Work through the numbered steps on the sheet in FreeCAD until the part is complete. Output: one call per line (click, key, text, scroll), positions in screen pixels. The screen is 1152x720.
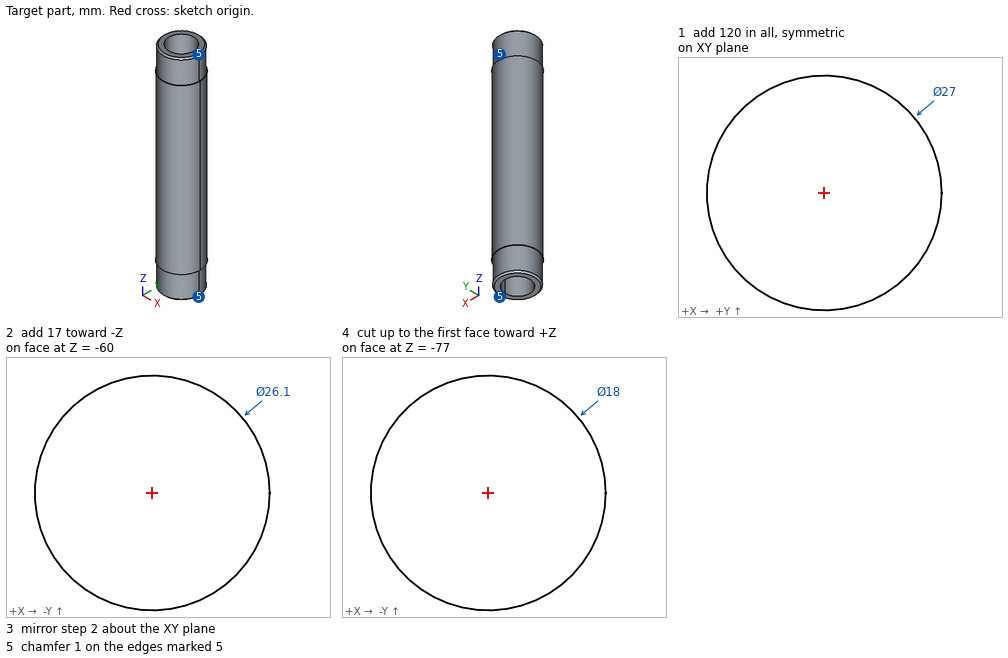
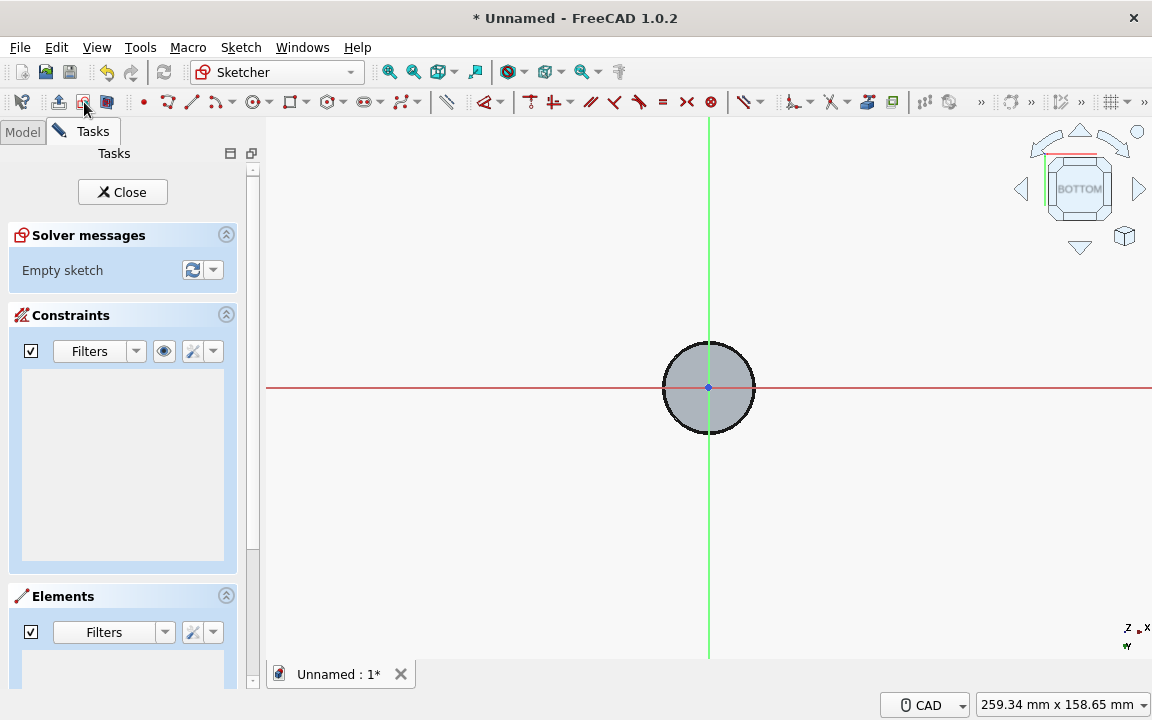
scroll(722, 388, up, 9)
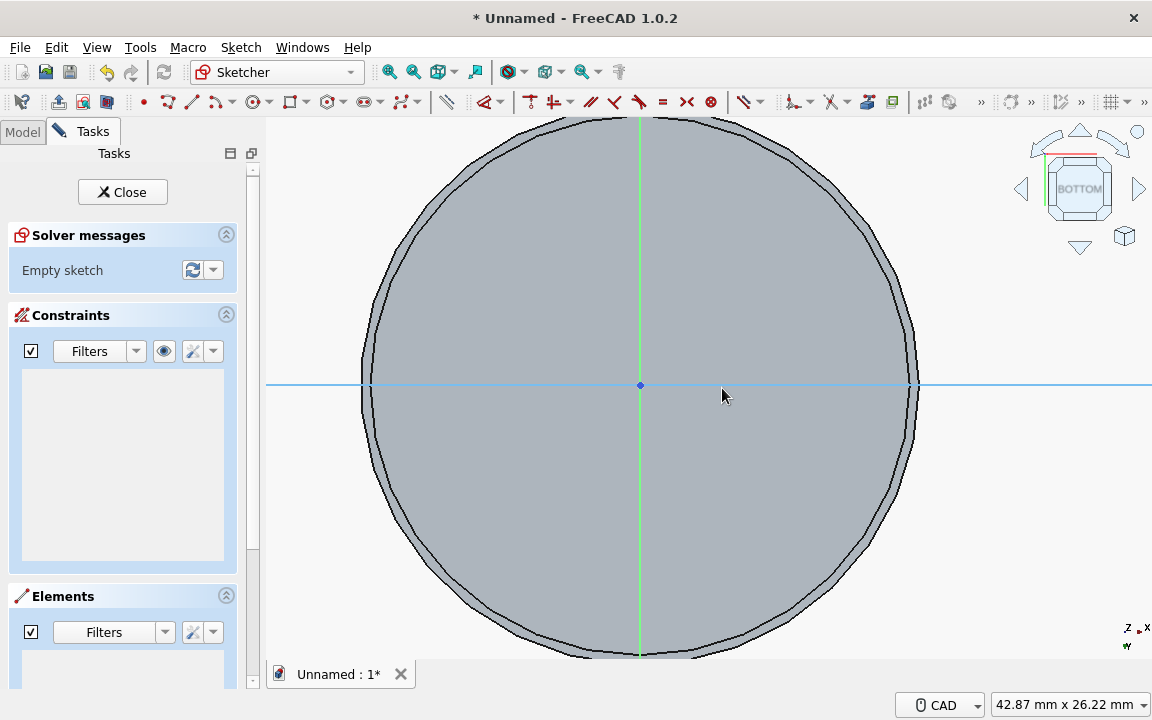
click(254, 102)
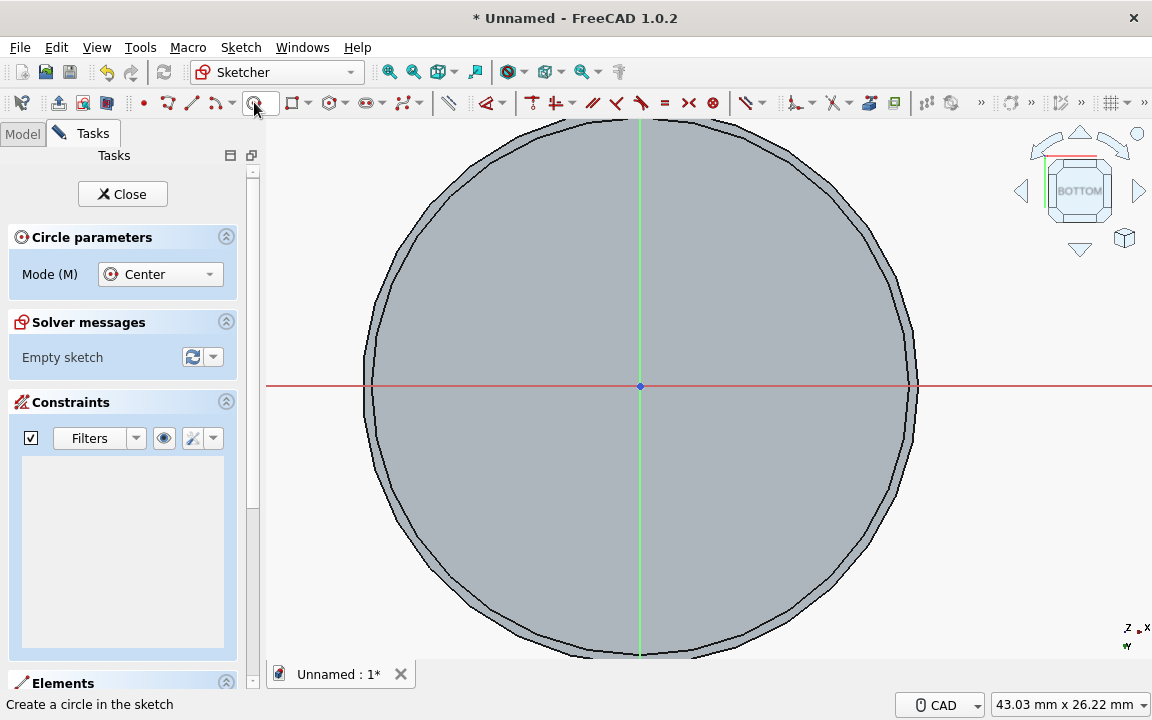
click(640, 386)
move(771, 255)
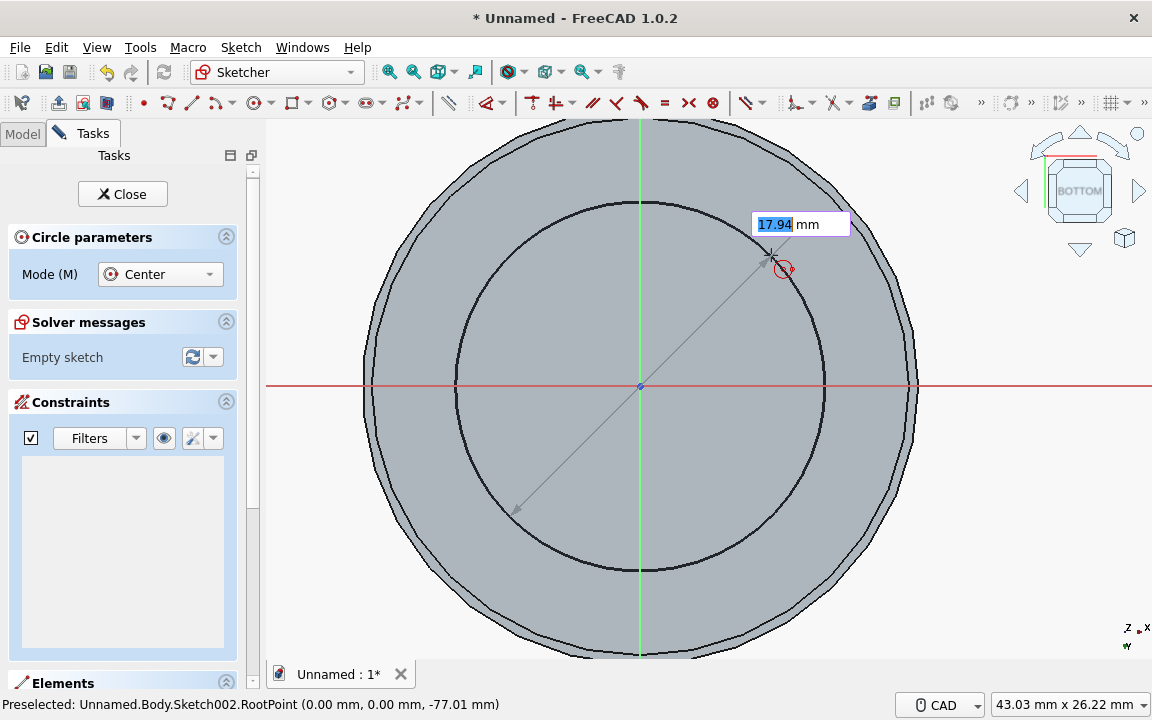
text(18)
key(Return)
key(Escape)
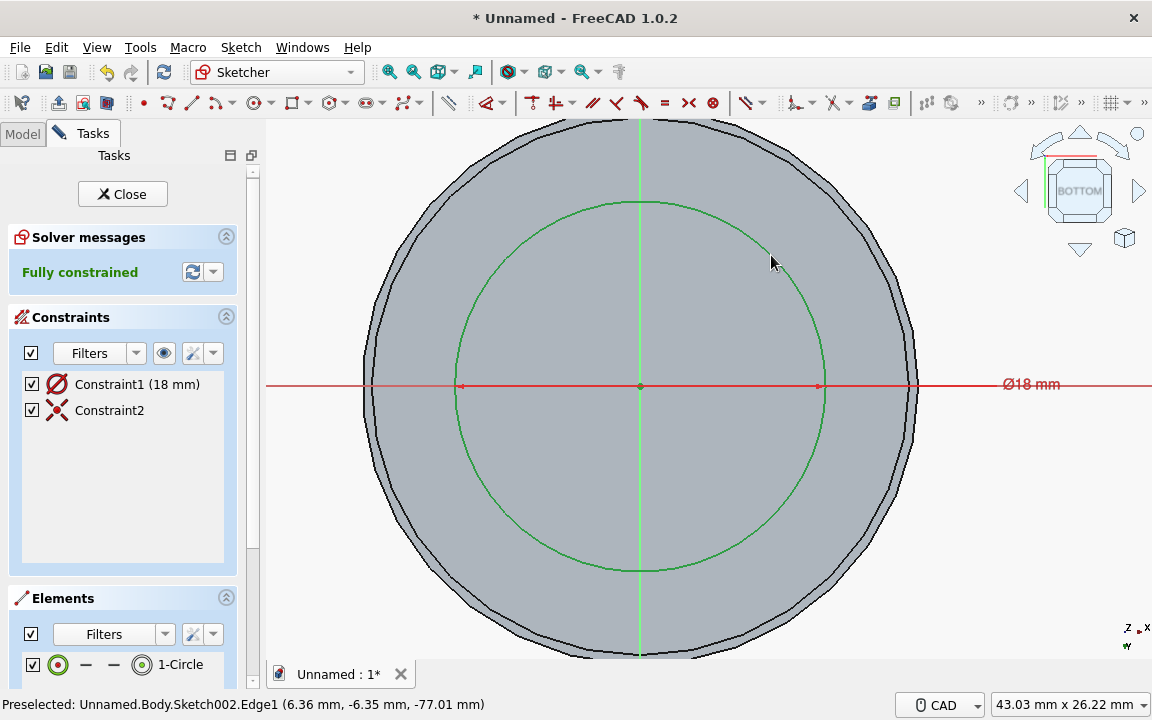
click(123, 194)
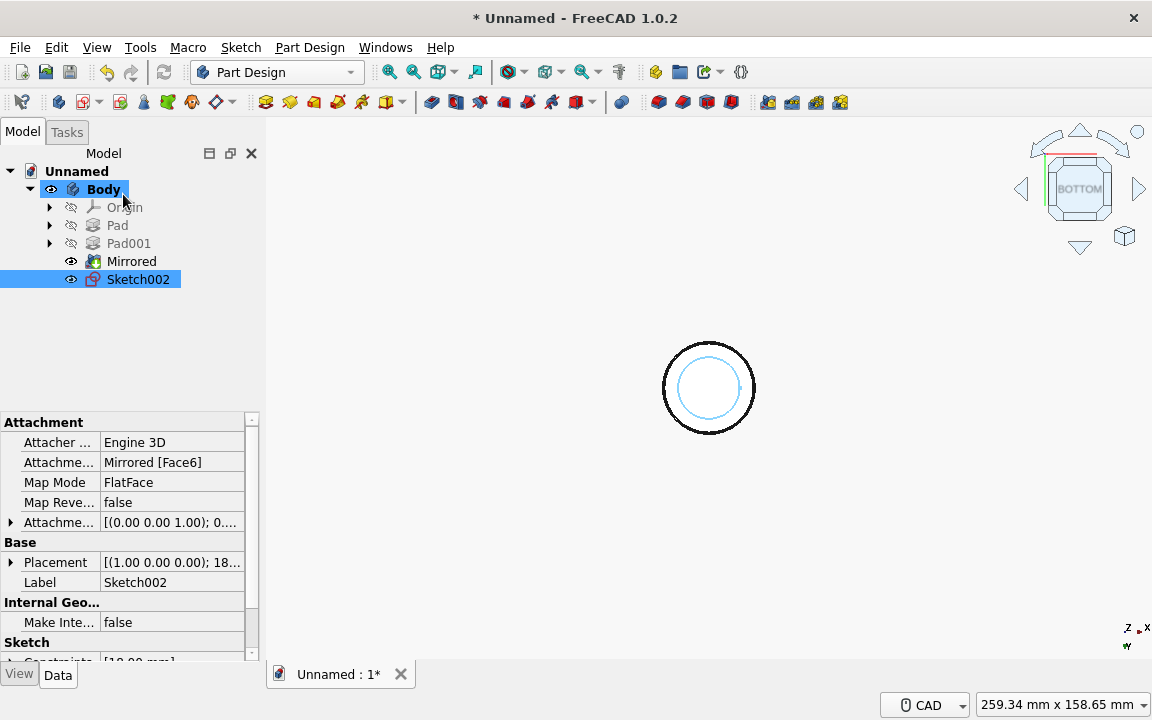
click(432, 102)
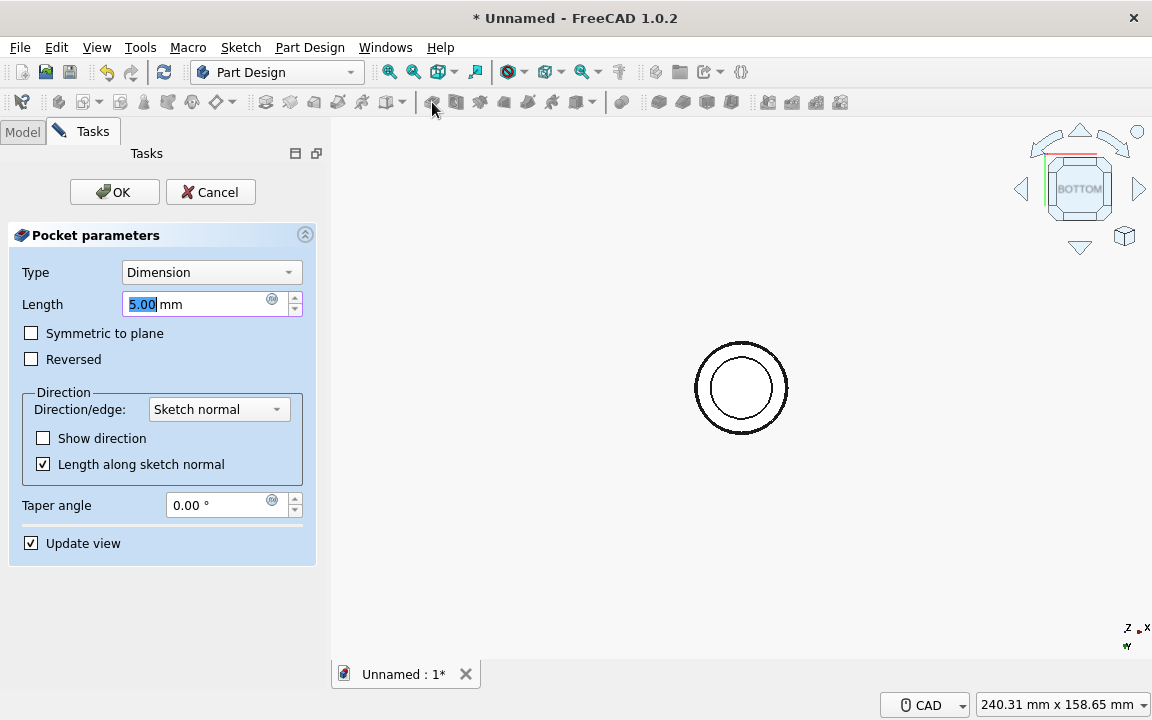
click(212, 272)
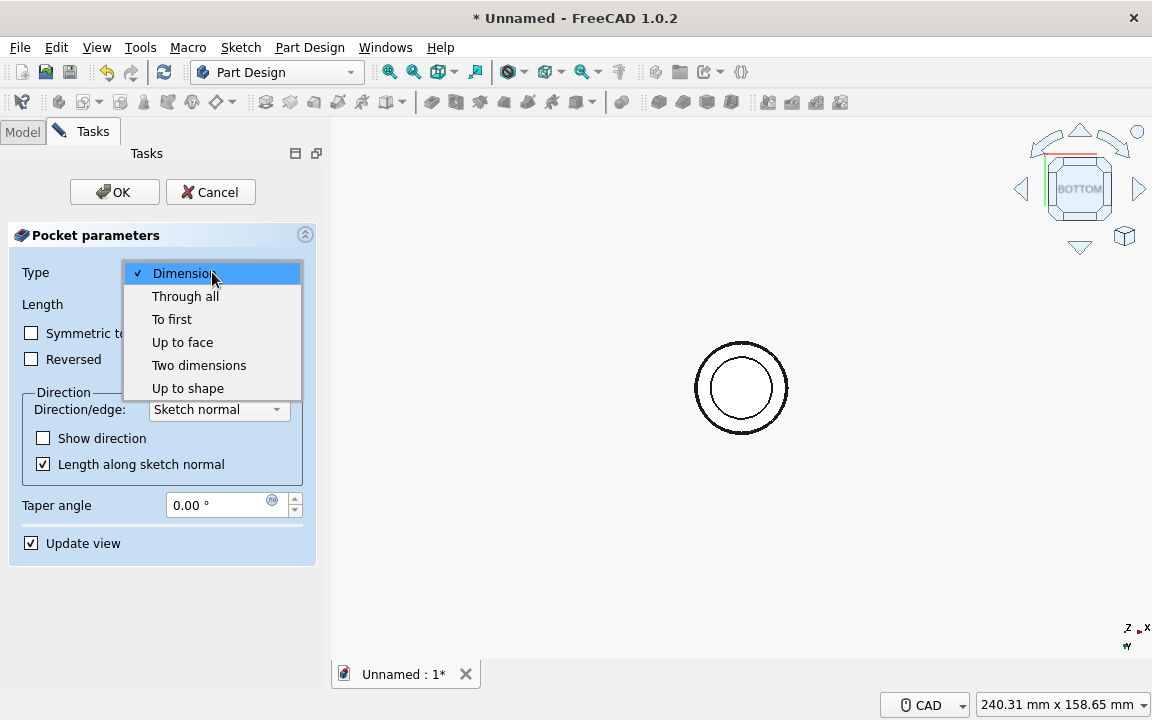
click(212, 320)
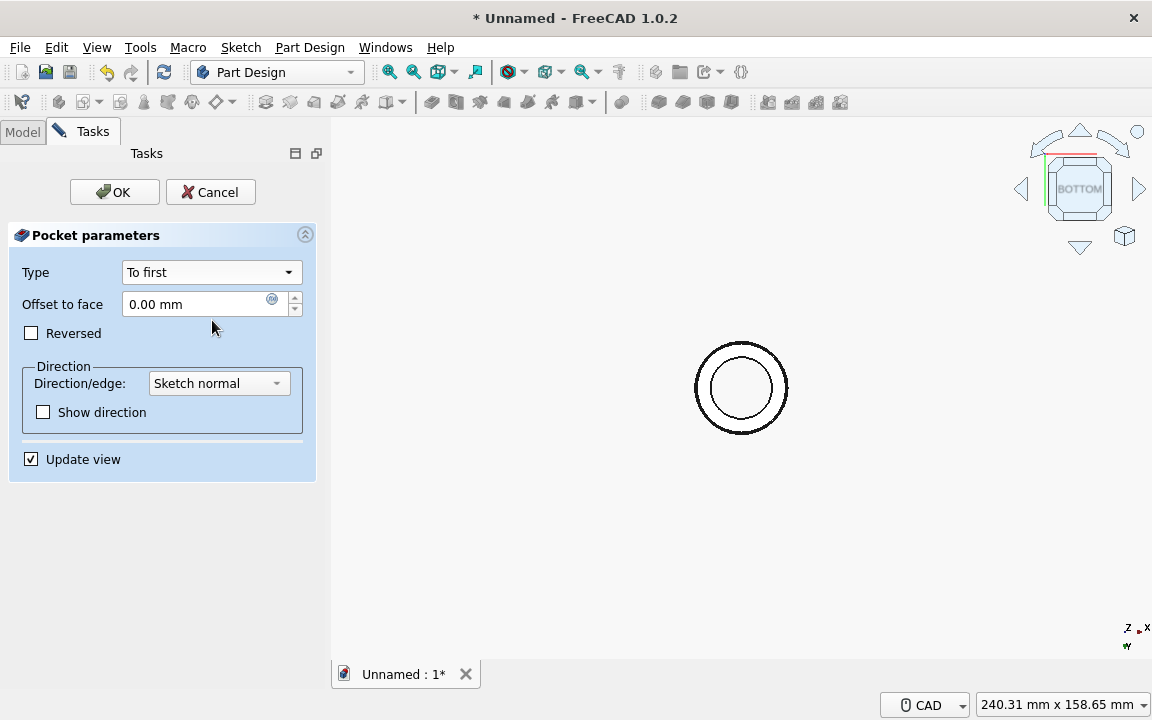
click(115, 192)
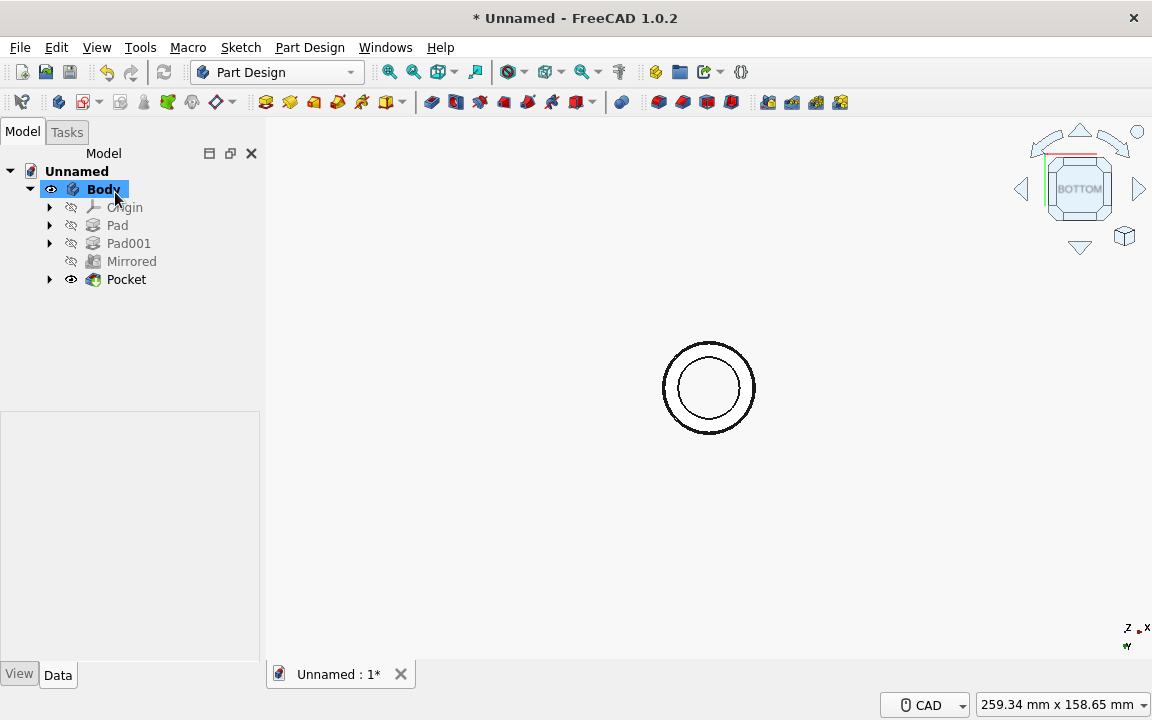
click(390, 72)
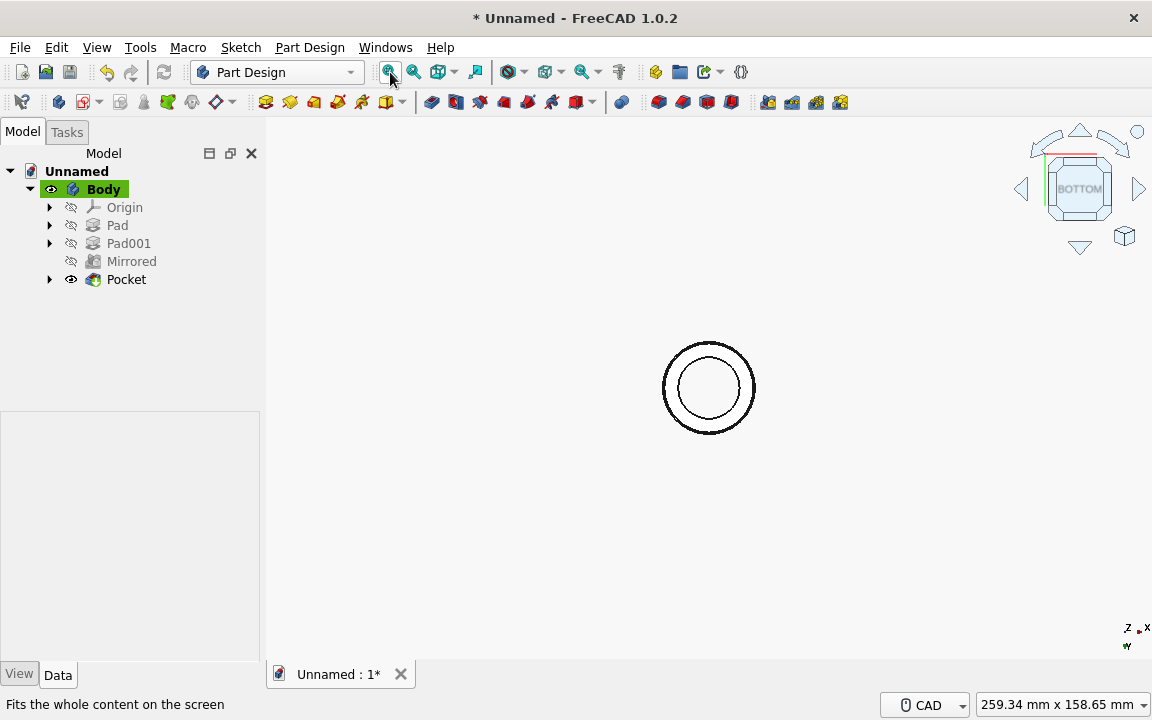
click(664, 387)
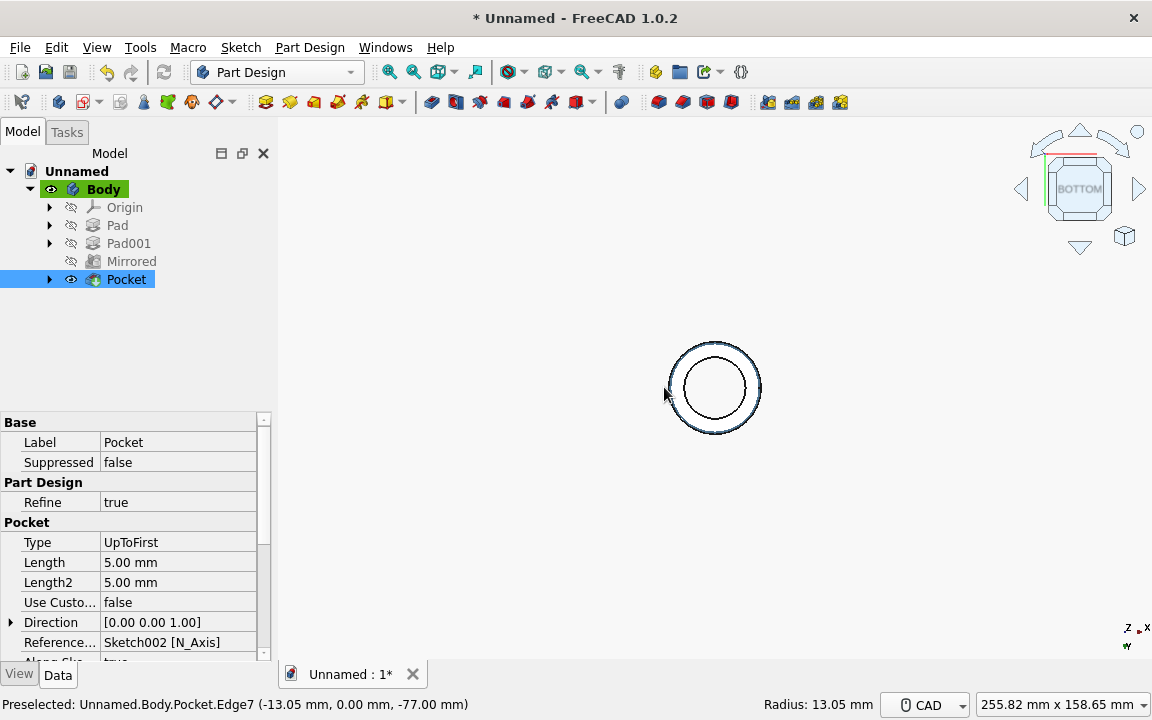
key(0)